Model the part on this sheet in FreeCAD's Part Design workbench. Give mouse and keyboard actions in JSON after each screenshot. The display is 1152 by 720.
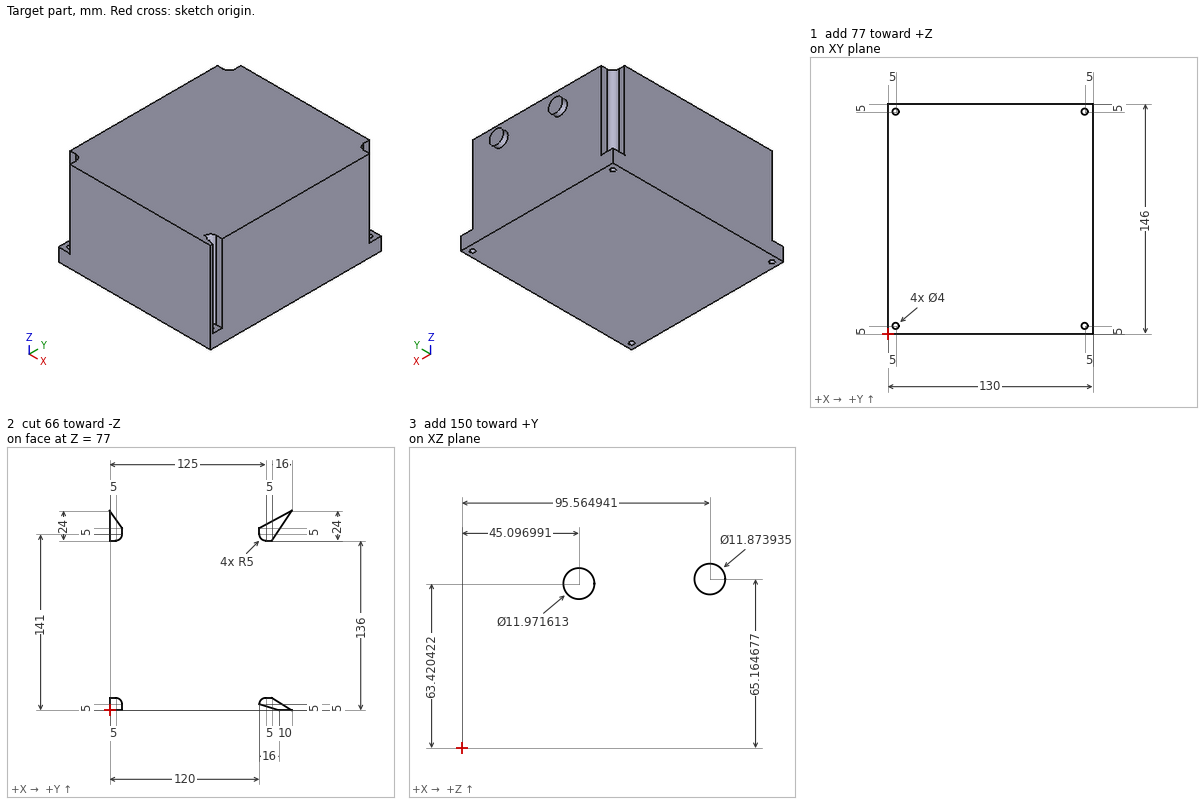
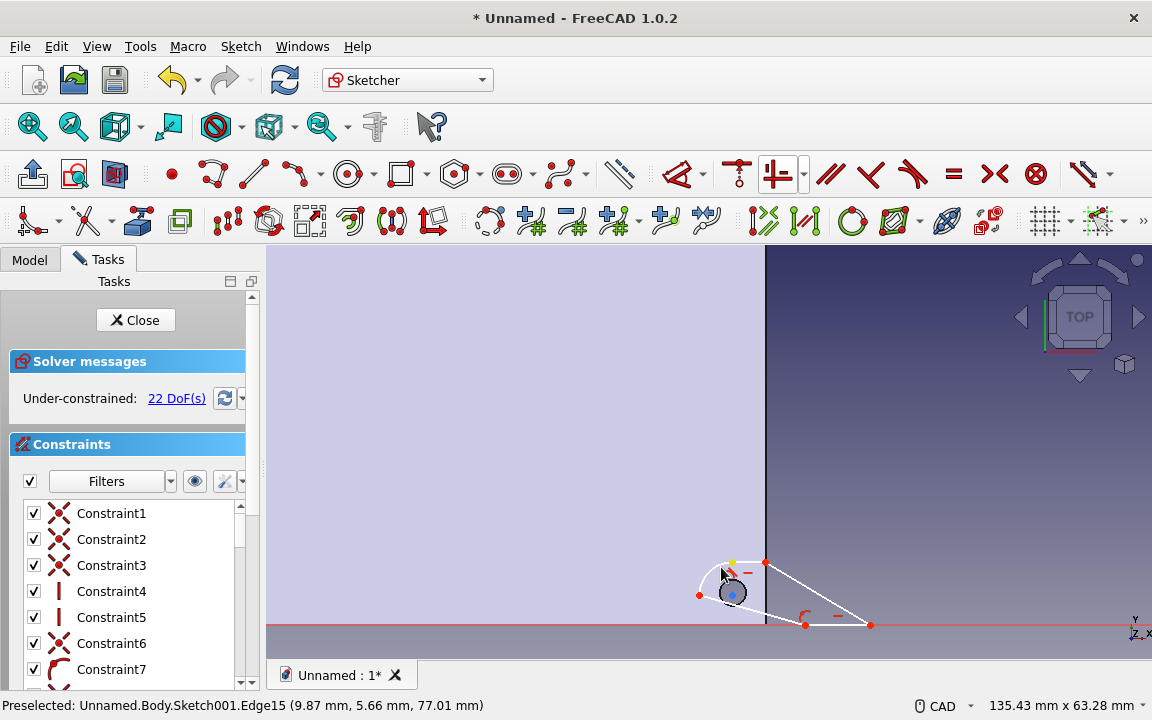
{"action": "left_click", "coordinate": [717, 566]}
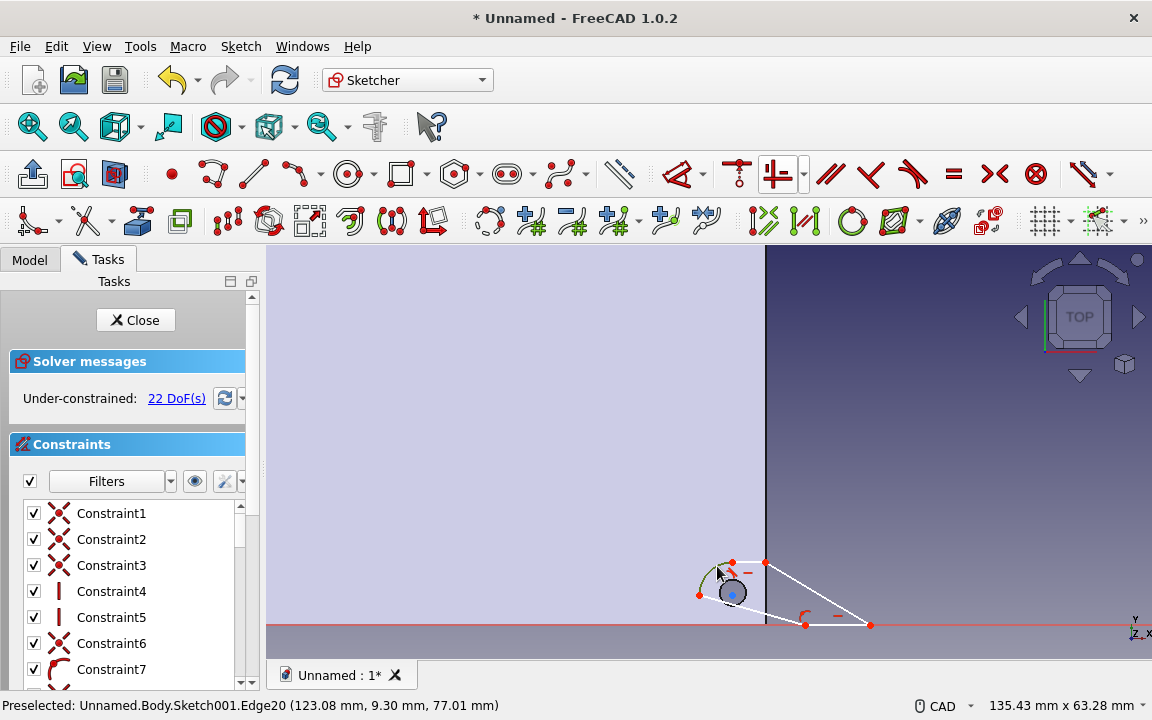
{"action": "left_click", "coordinate": [954, 174]}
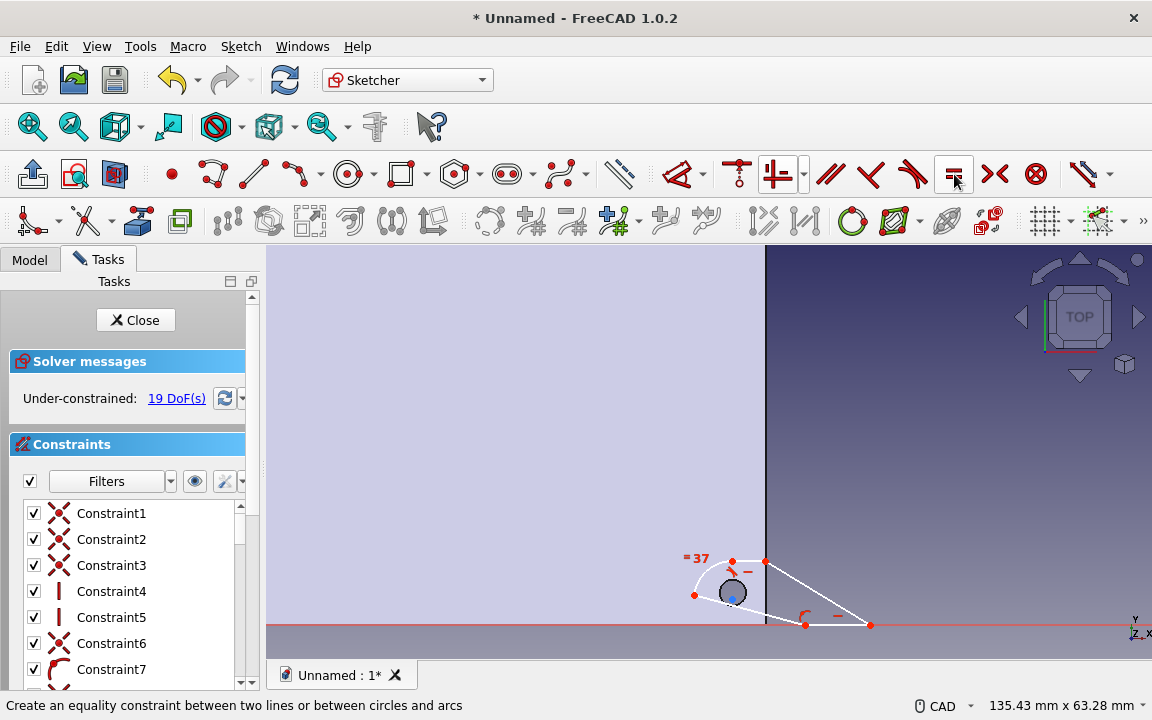
{"action": "left_click", "coordinate": [676, 174]}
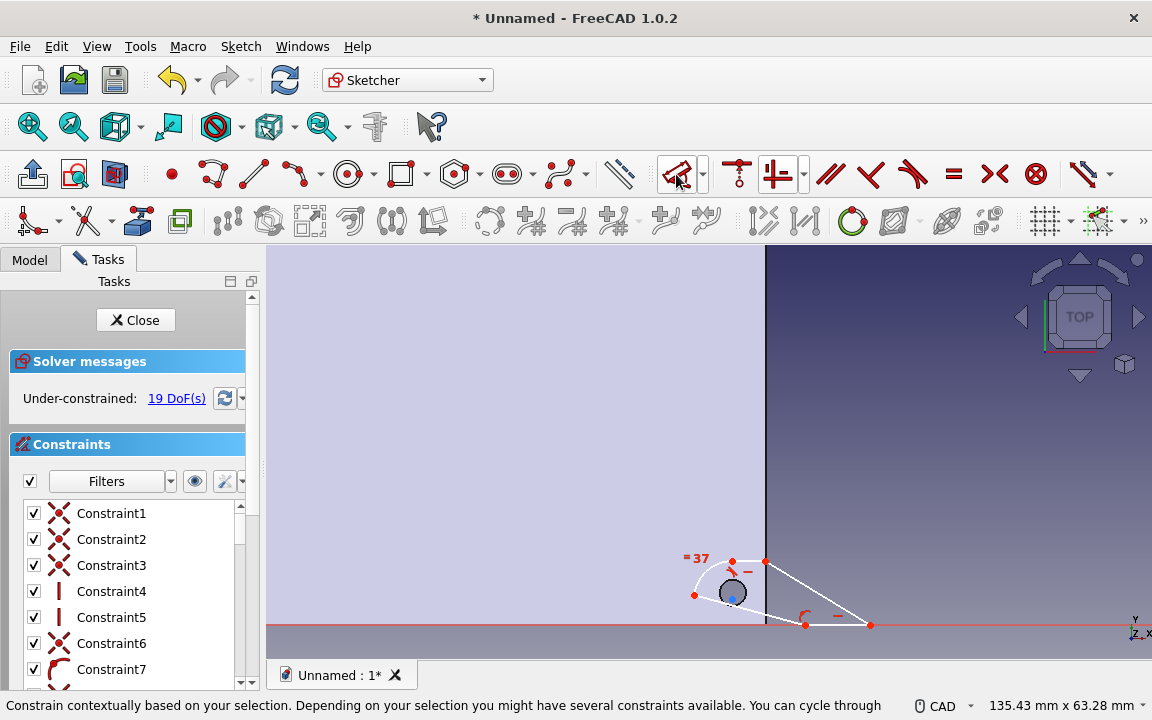
{"action": "scroll", "coordinate": [722, 567], "scroll_direction": "down", "scroll_amount": 7}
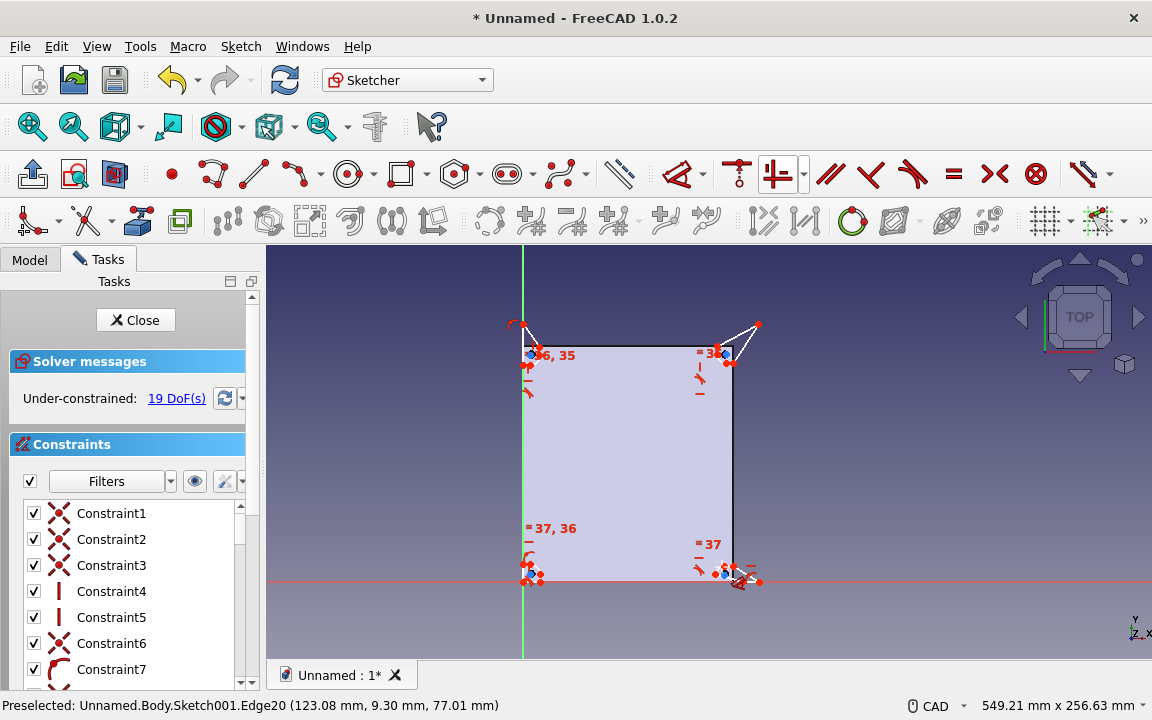
{"action": "scroll", "coordinate": [718, 358], "scroll_direction": "up", "scroll_amount": 8}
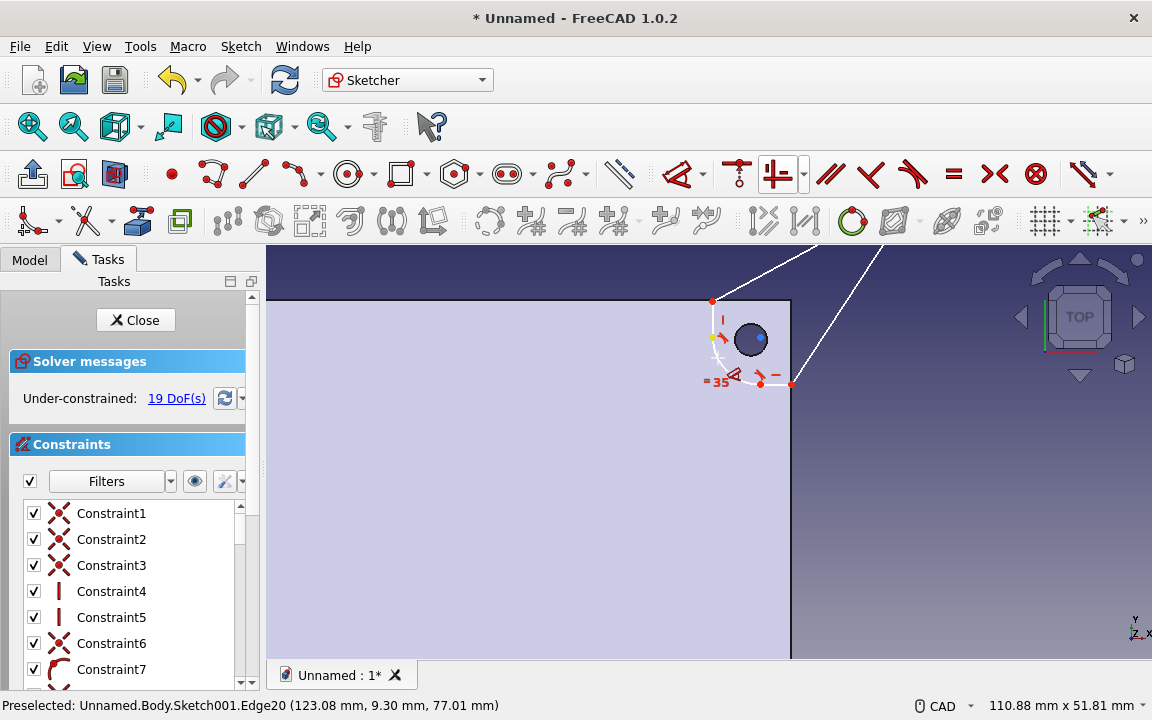
{"action": "left_click", "coordinate": [718, 359]}
{"action": "left_click", "coordinate": [690, 374]}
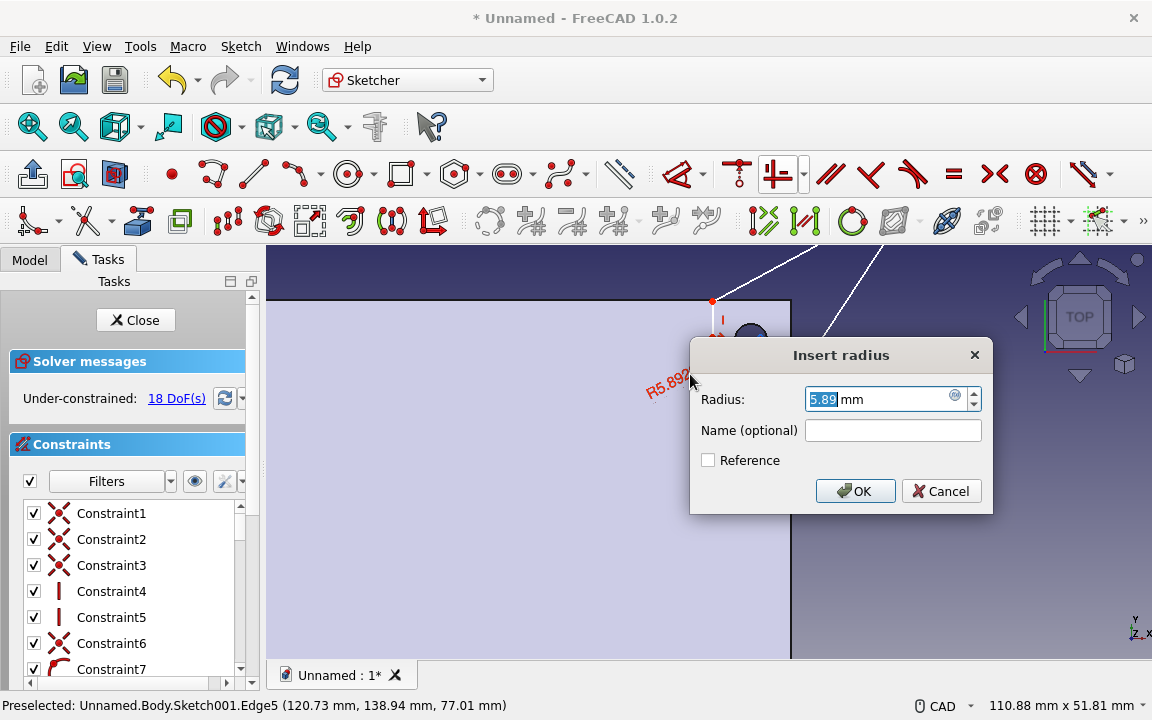
{"action": "type", "text": "5"}
{"action": "key", "text": "Return"}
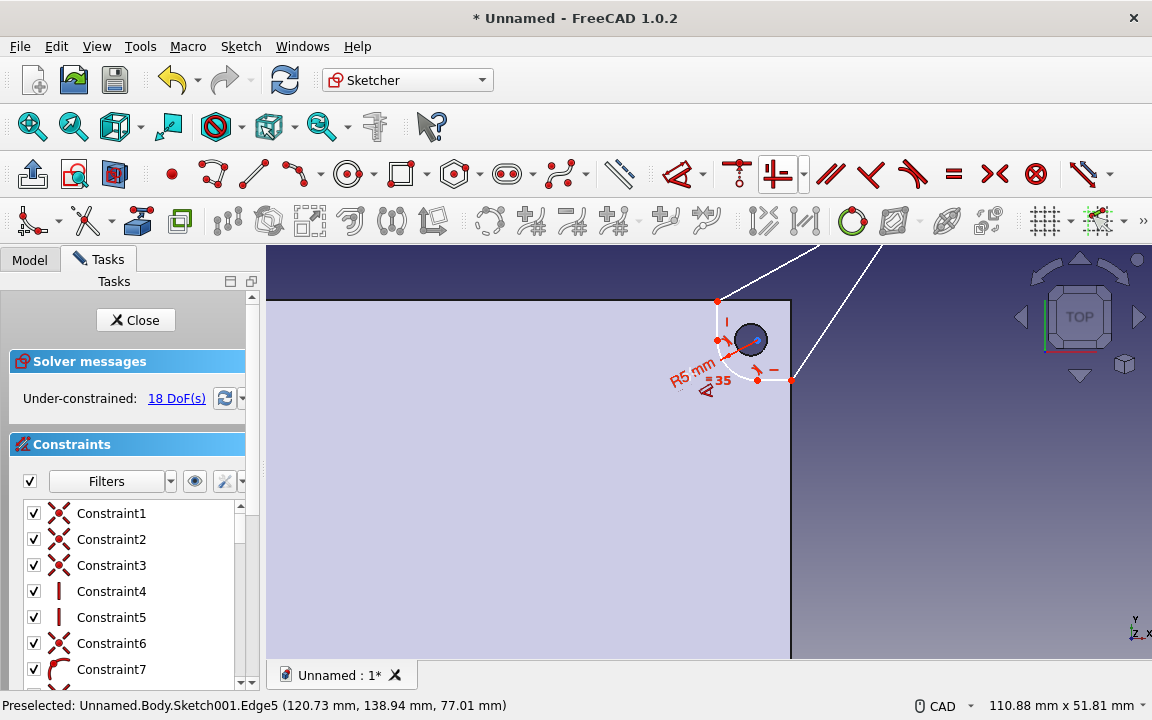
{"action": "scroll", "coordinate": [768, 380], "scroll_direction": "up", "scroll_amount": 2}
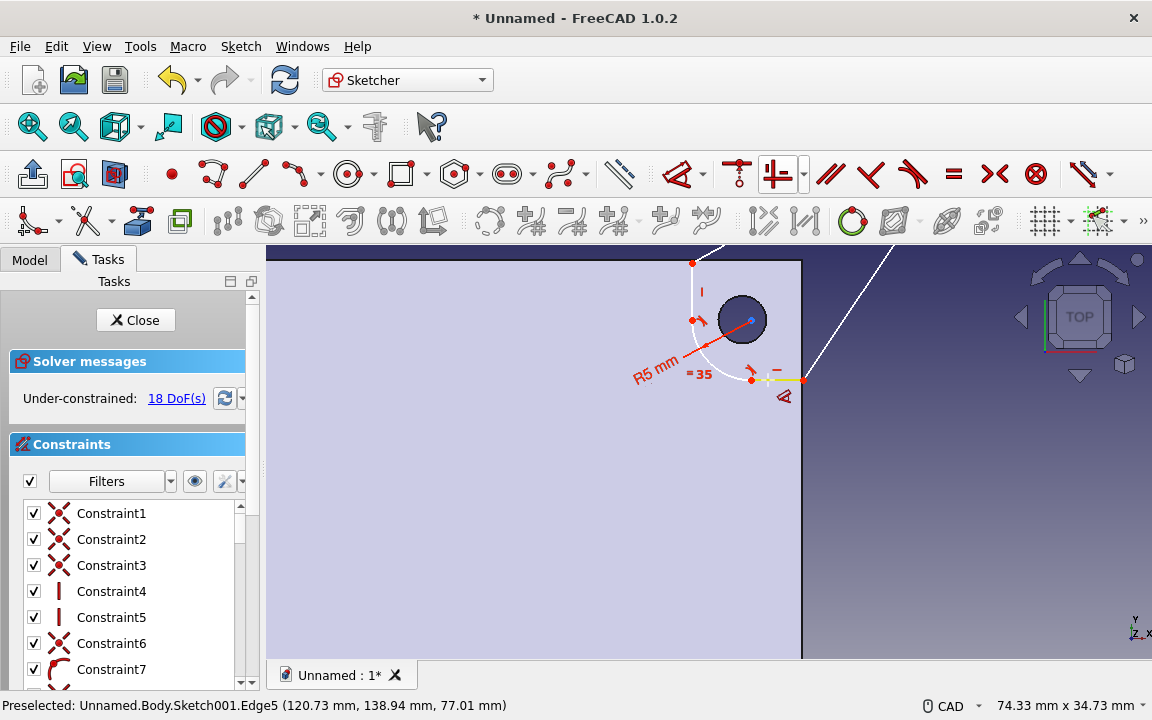
{"action": "left_click", "coordinate": [767, 380]}
{"action": "left_click", "coordinate": [778, 346]}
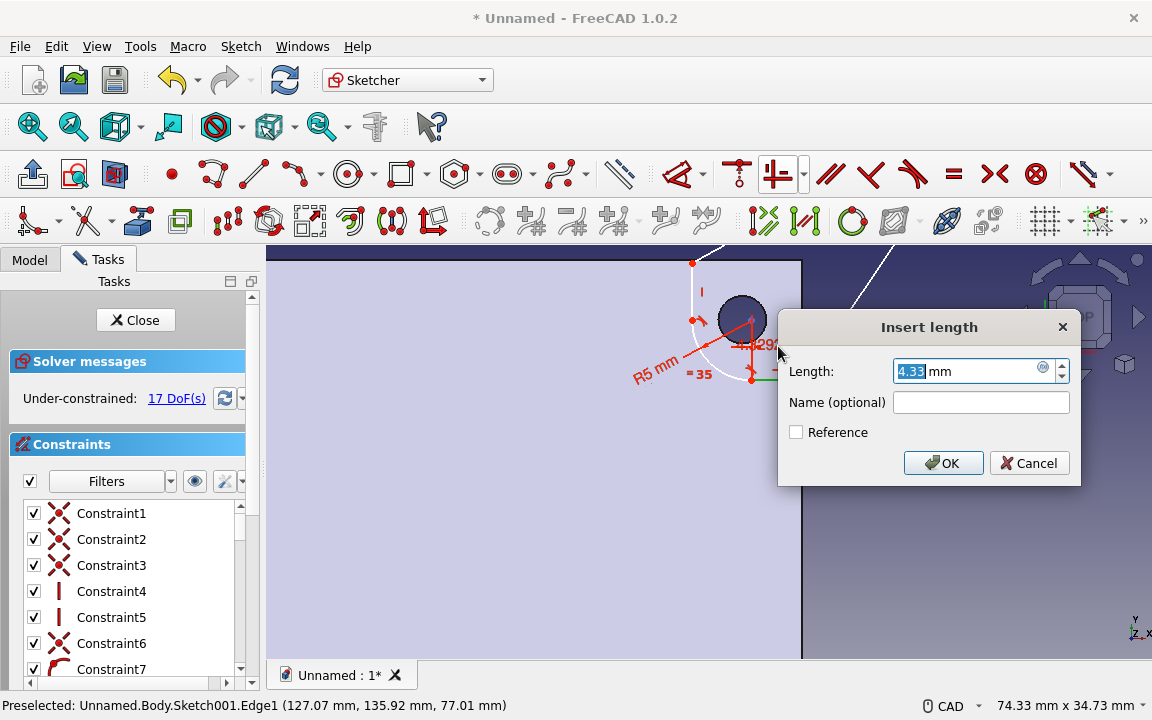
{"action": "type", "text": "5"}
{"action": "key", "text": "Return"}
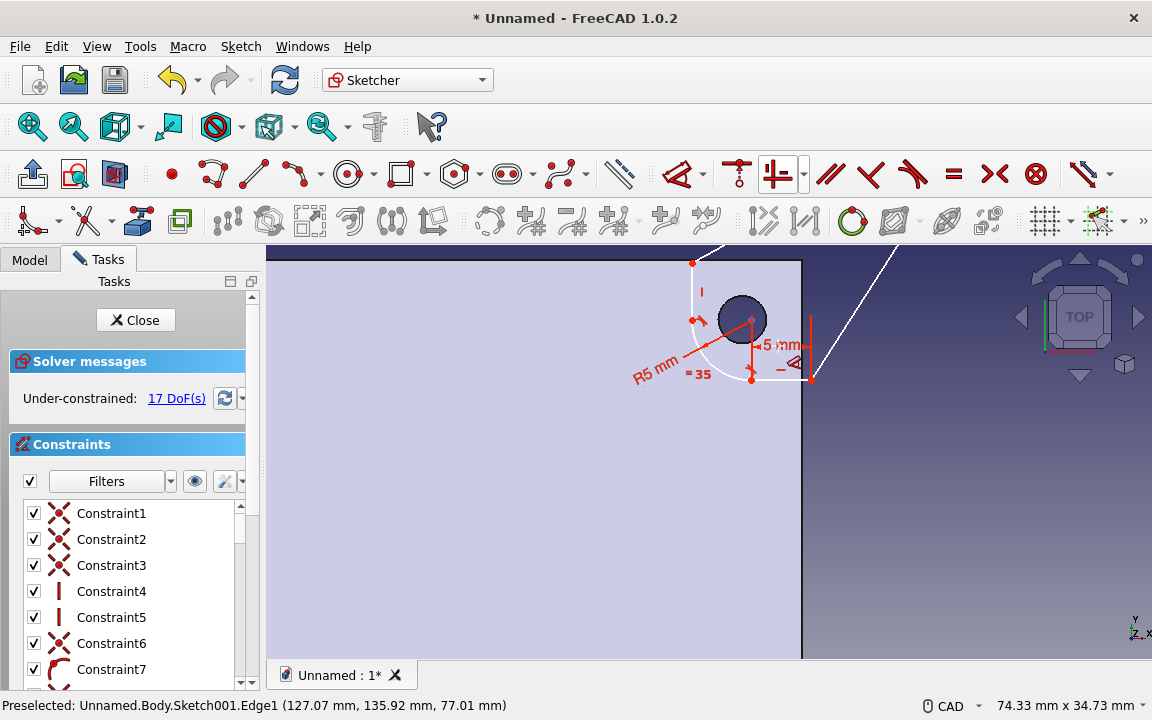
{"action": "left_click", "coordinate": [692, 280]}
{"action": "left_click", "coordinate": [726, 297]}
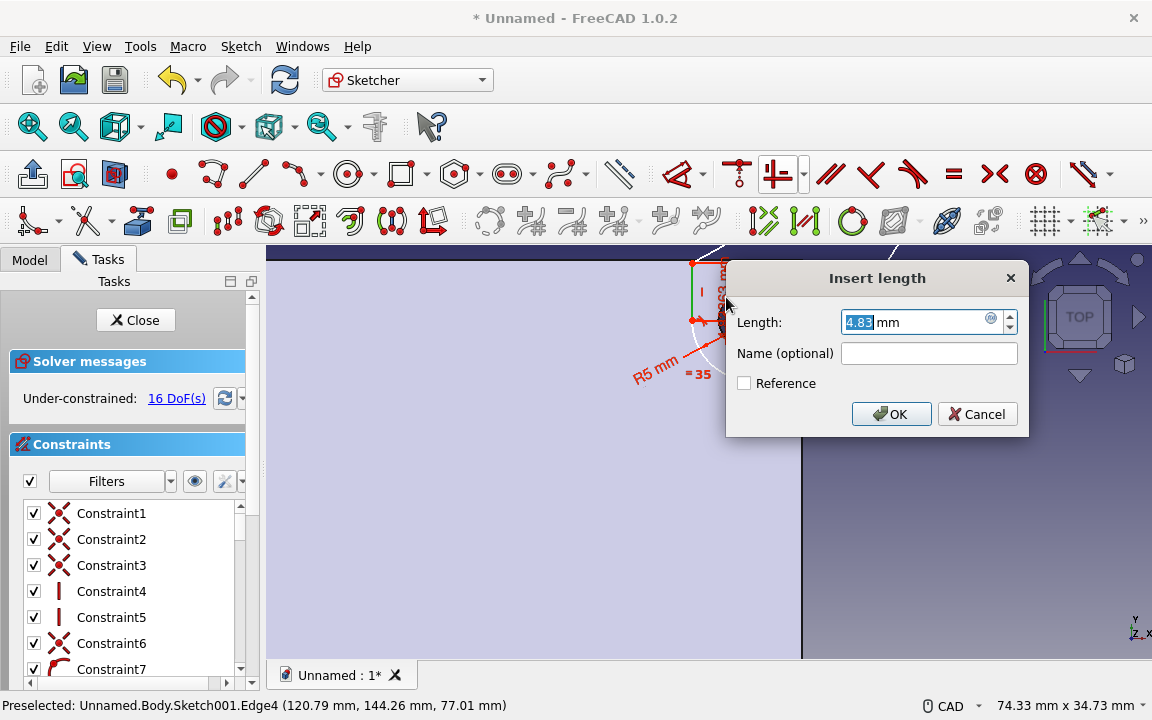
{"action": "type", "text": "5"}
{"action": "key", "text": "Return"}